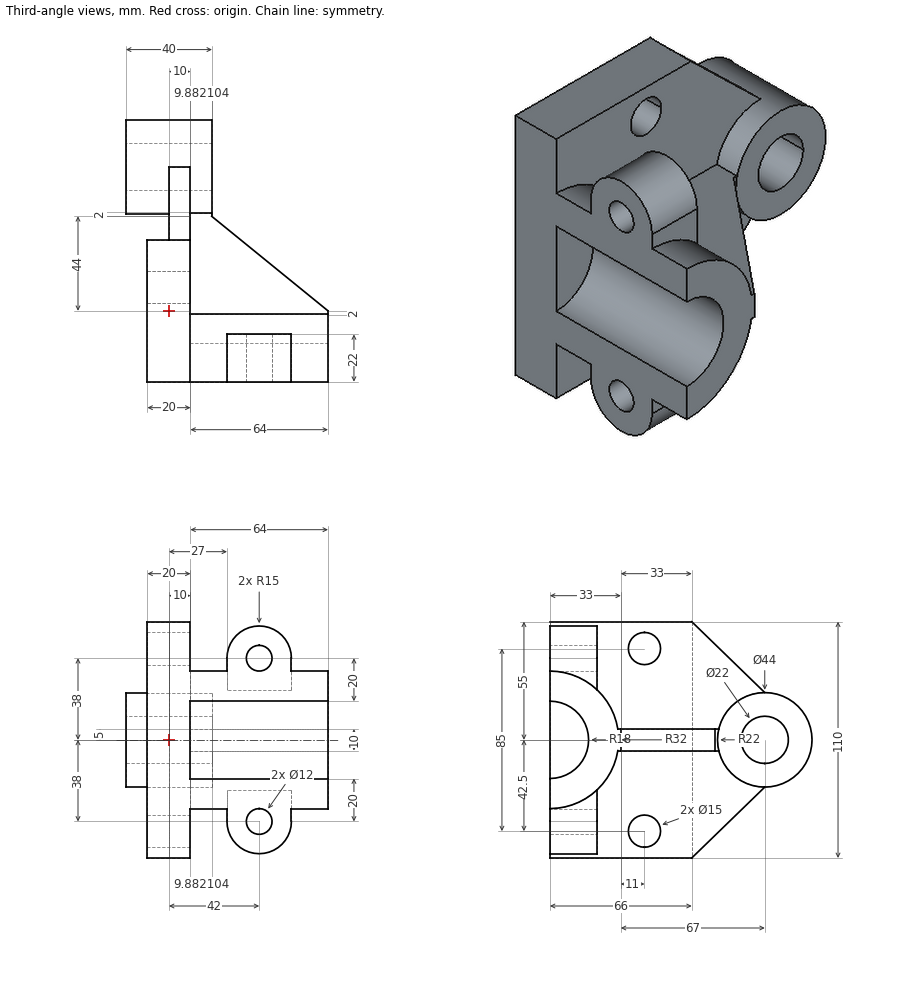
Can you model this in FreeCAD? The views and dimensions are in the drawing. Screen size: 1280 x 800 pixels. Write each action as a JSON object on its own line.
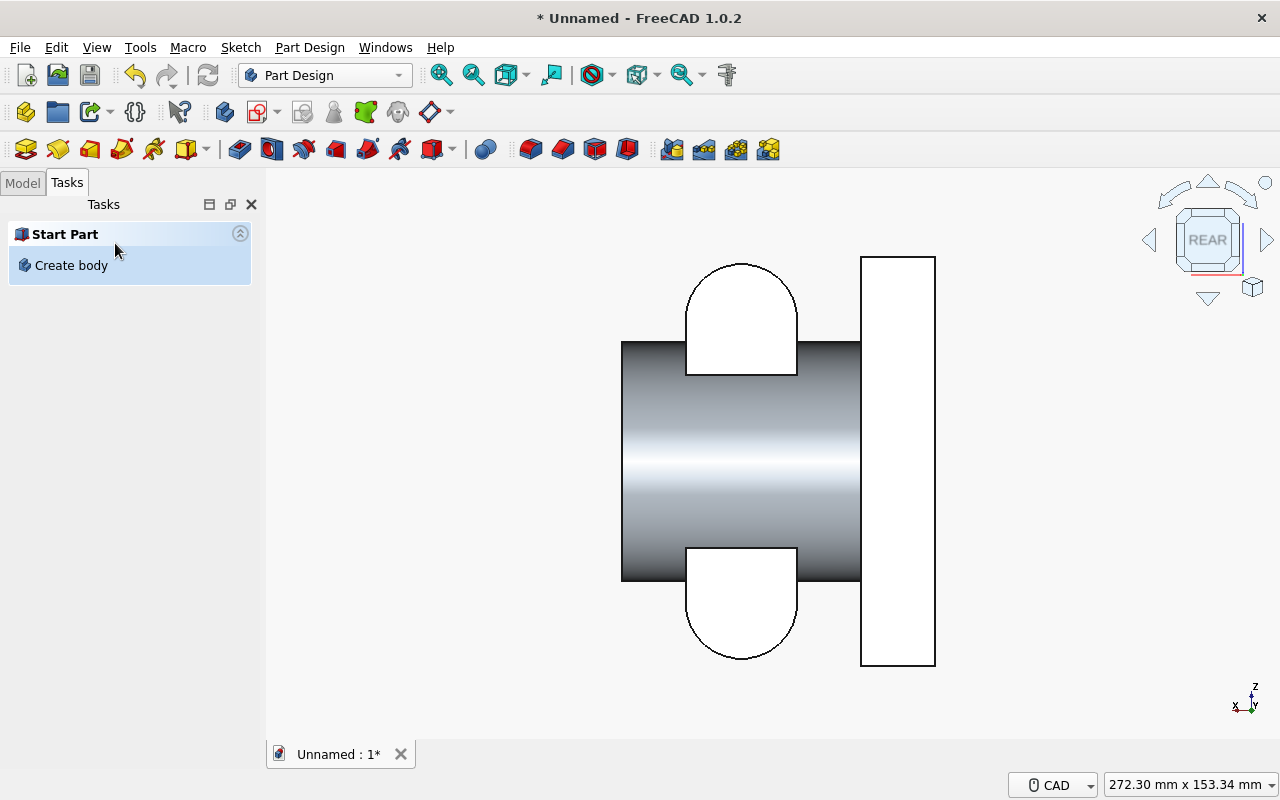
{"action": "left_click", "coordinate": [741, 602]}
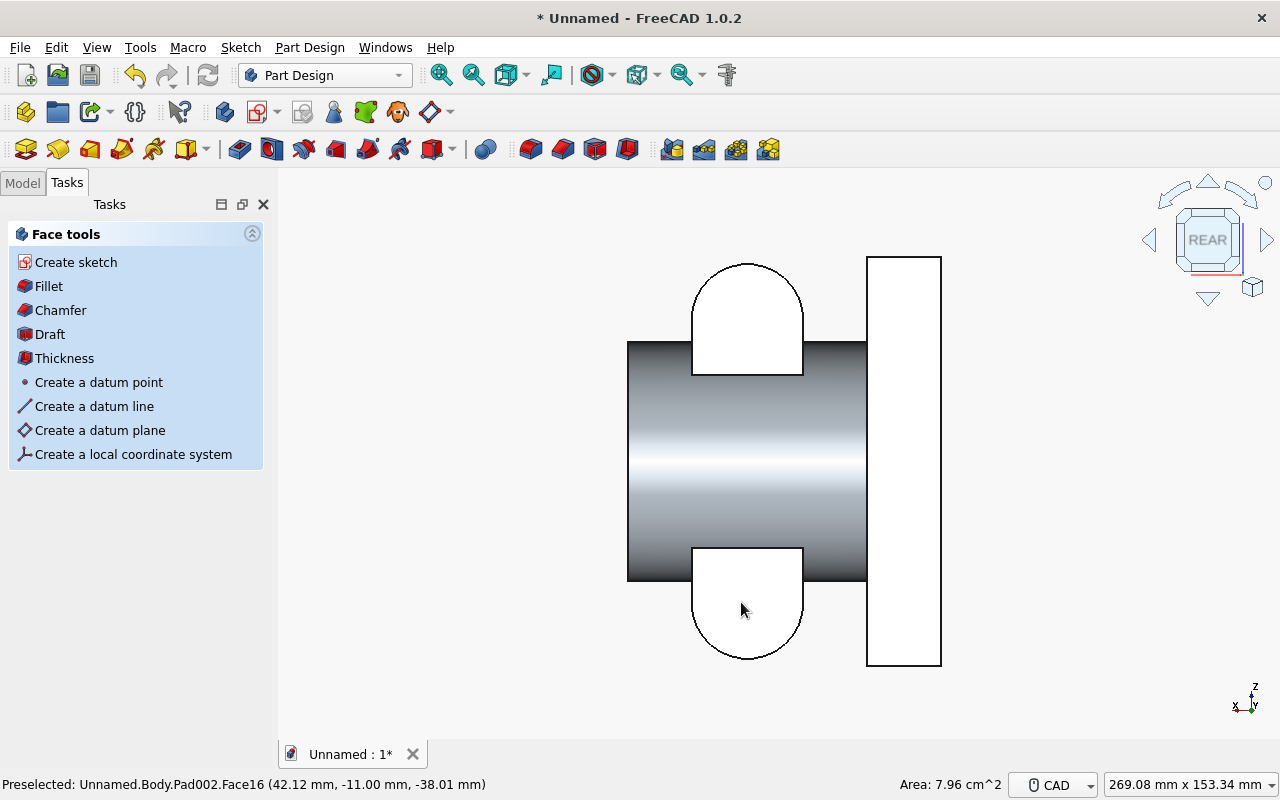
{"action": "left_click", "coordinate": [258, 112]}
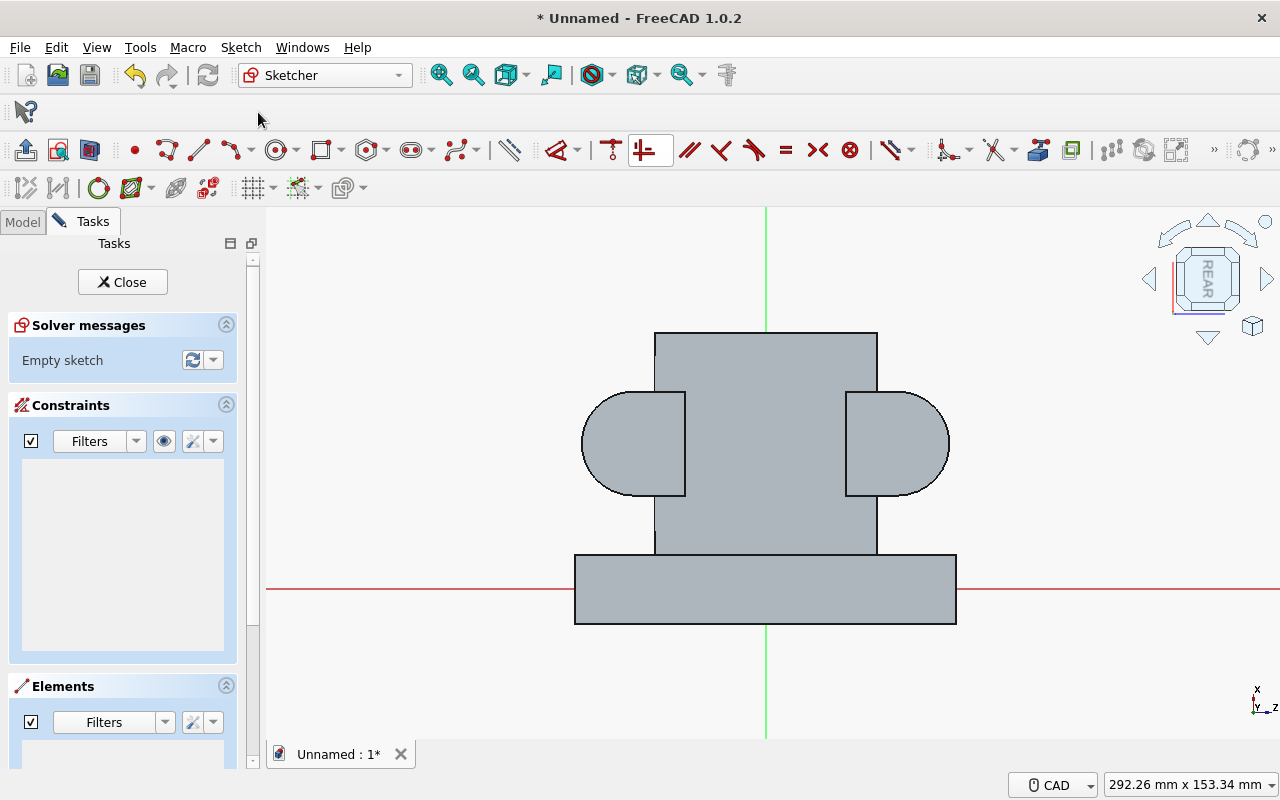
{"action": "left_click", "coordinate": [90, 150]}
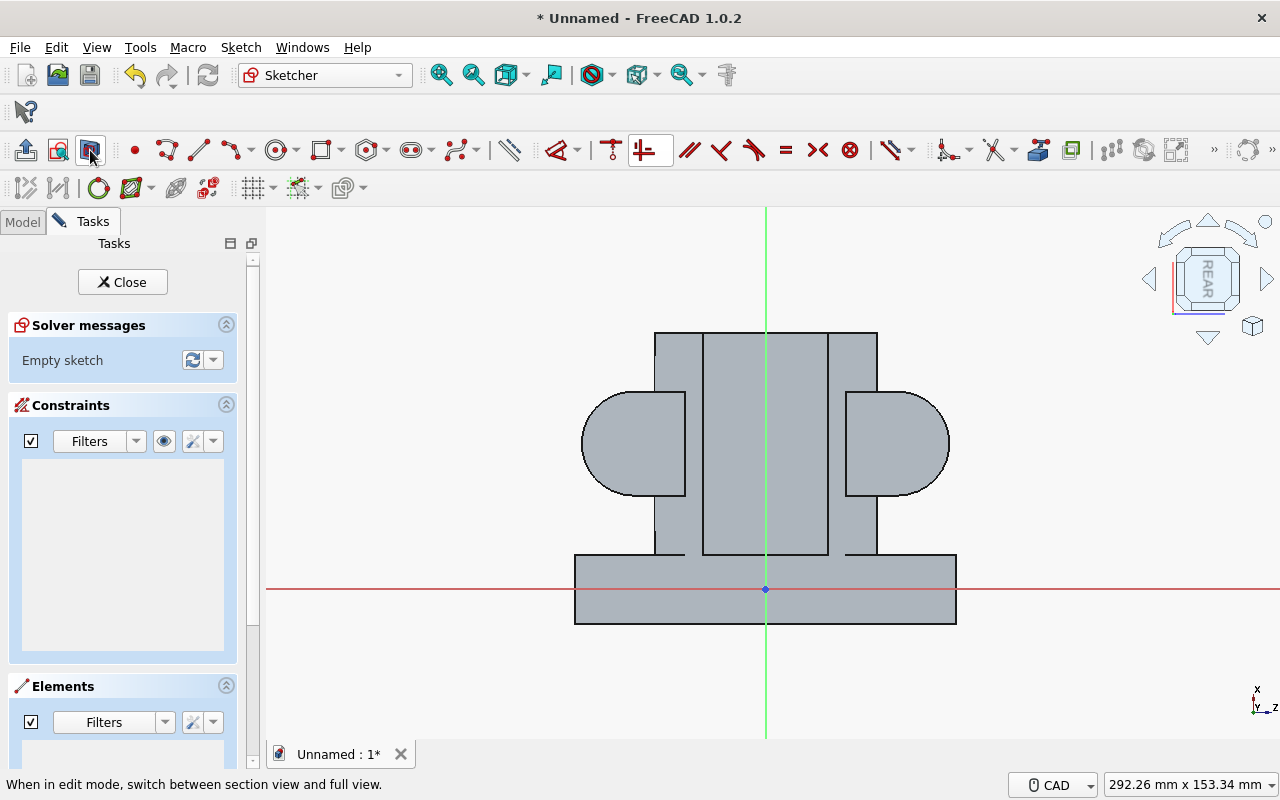
{"action": "scroll", "coordinate": [840, 546], "scroll_direction": "up", "scroll_amount": 3}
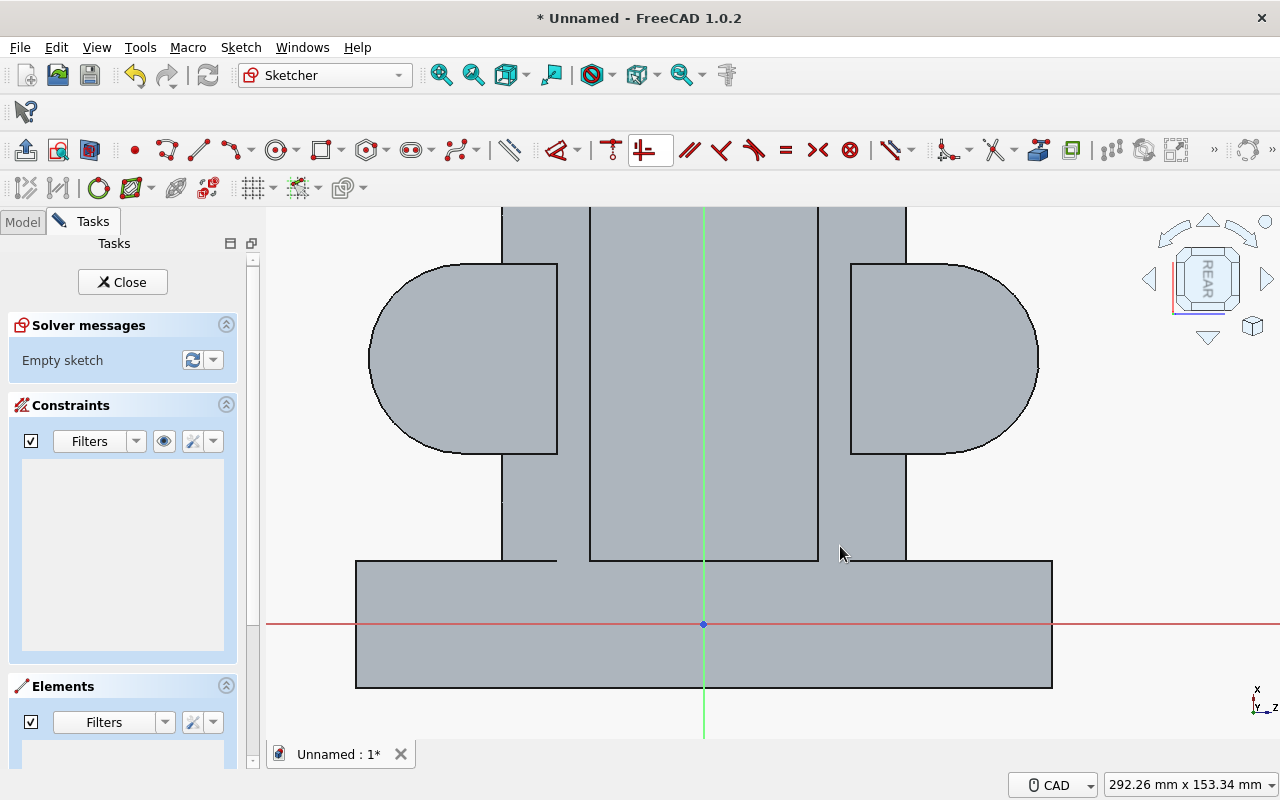
{"action": "left_click", "coordinate": [276, 150]}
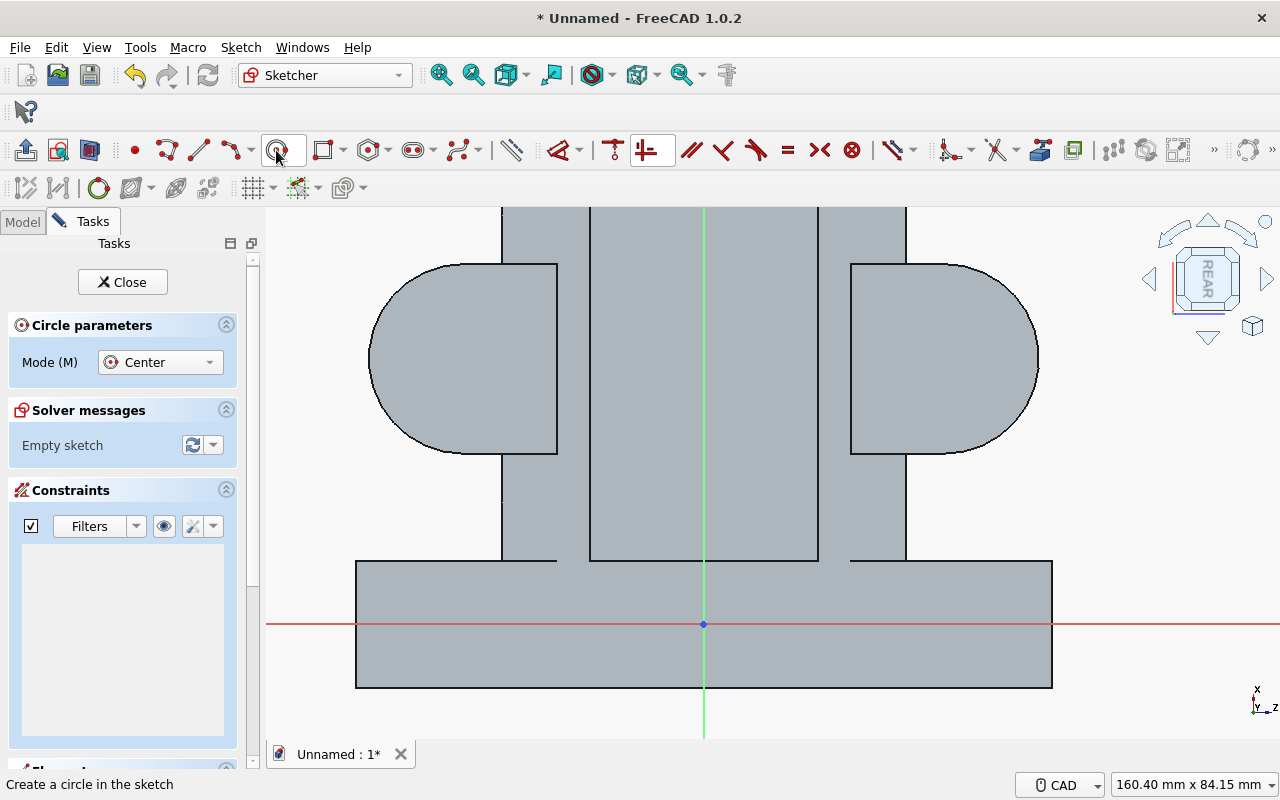
{"action": "left_click", "coordinate": [464, 359]}
{"action": "left_click", "coordinate": [491, 332]}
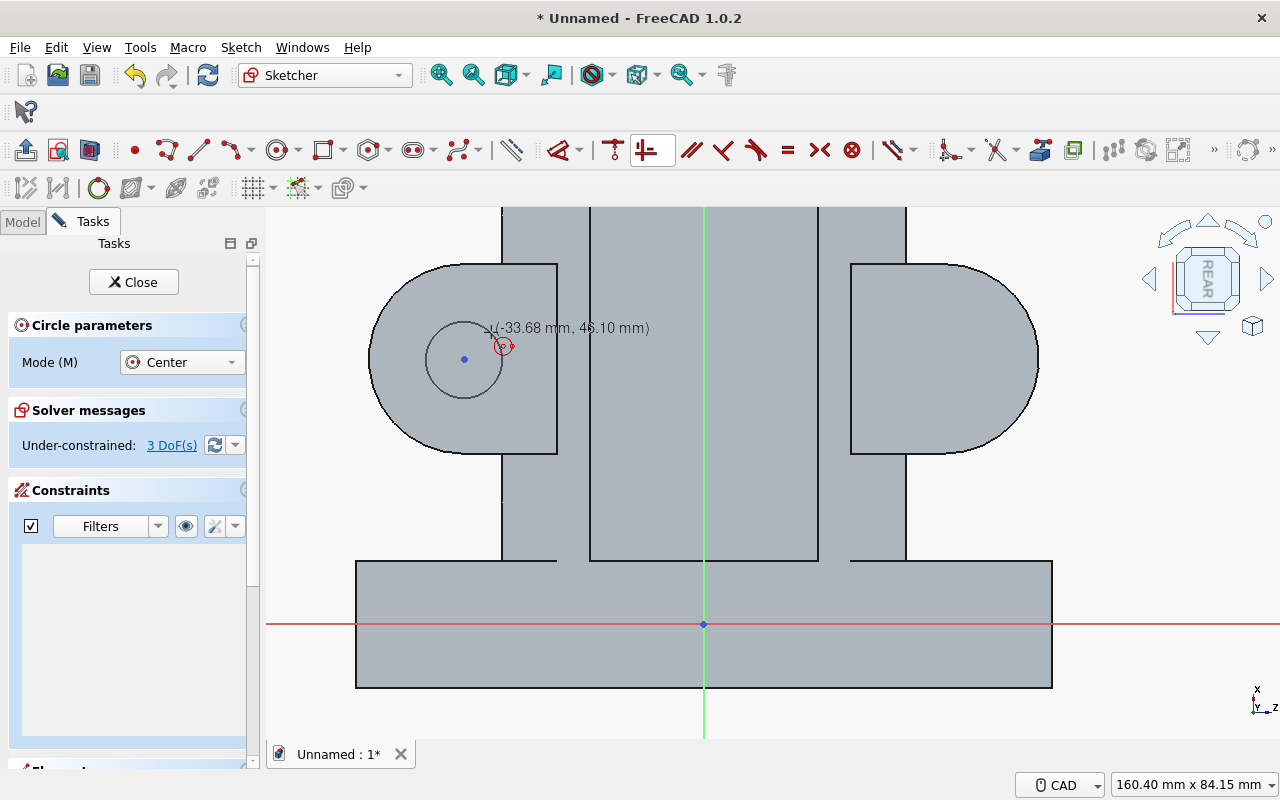
{"action": "left_click", "coordinate": [944, 359]}
{"action": "left_click", "coordinate": [971, 332]}
{"action": "key", "text": "Escape"}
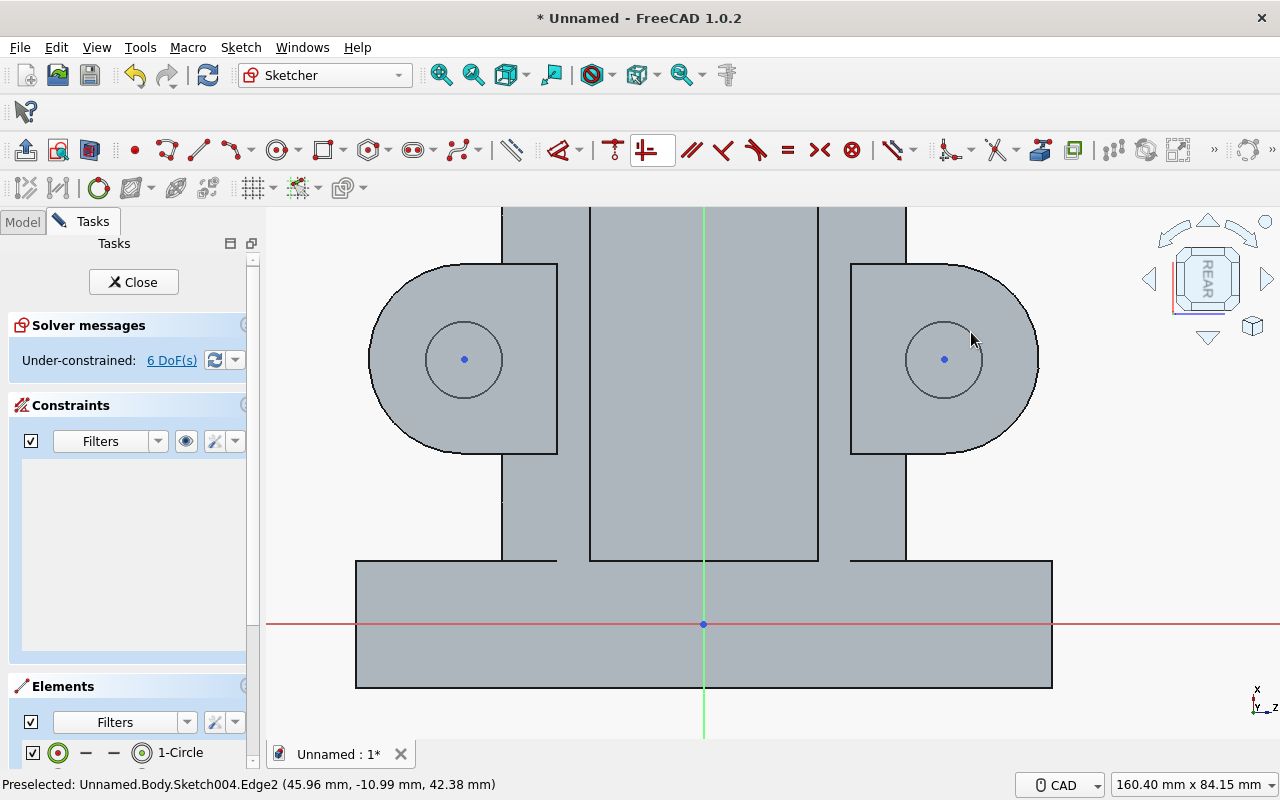
{"action": "left_click", "coordinate": [491, 333]}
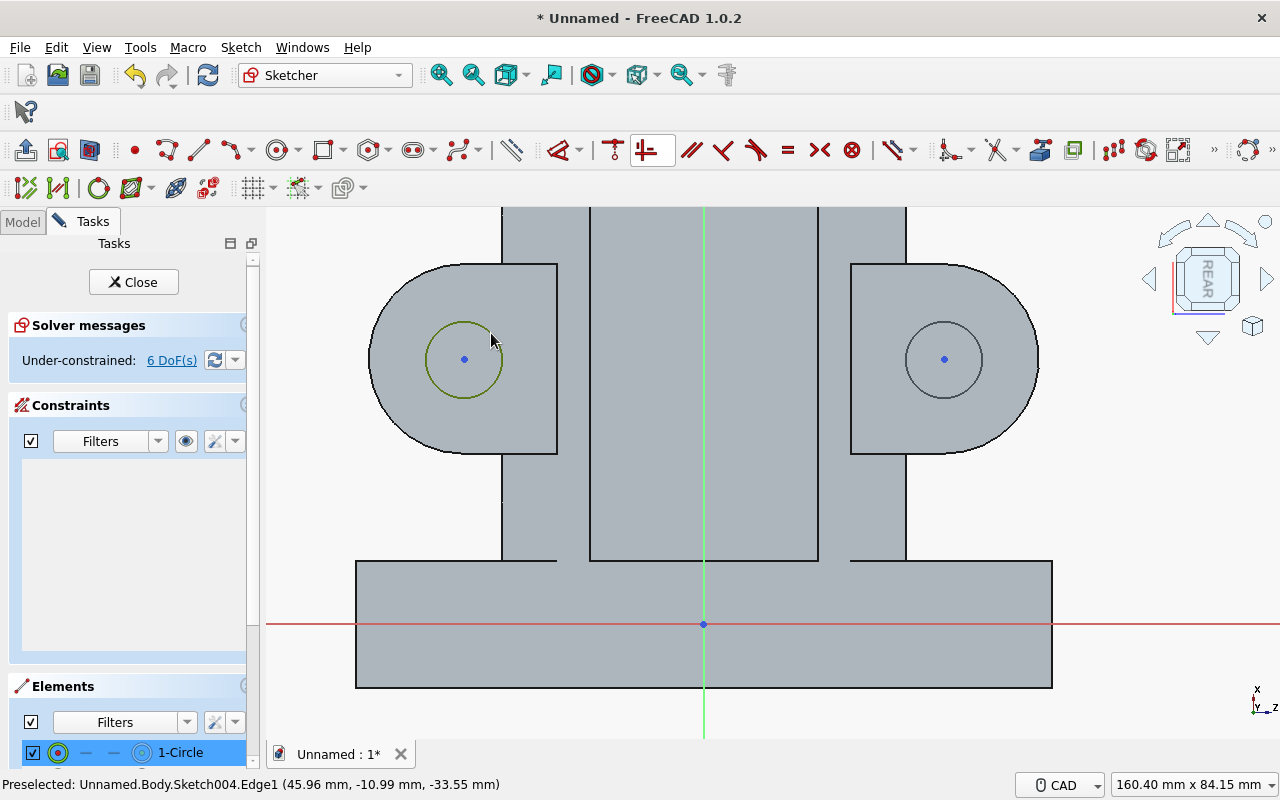
{"action": "left_click", "coordinate": [971, 333]}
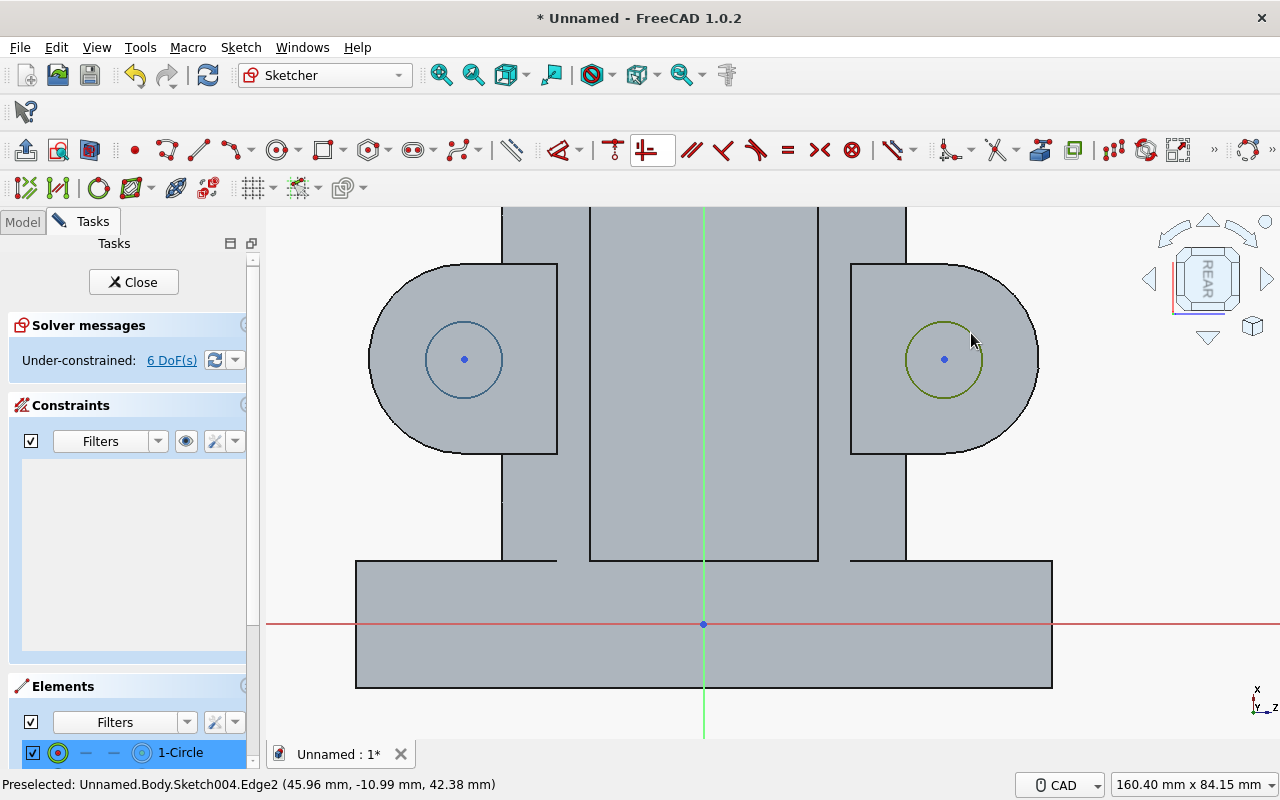
{"action": "key", "text": "e"}